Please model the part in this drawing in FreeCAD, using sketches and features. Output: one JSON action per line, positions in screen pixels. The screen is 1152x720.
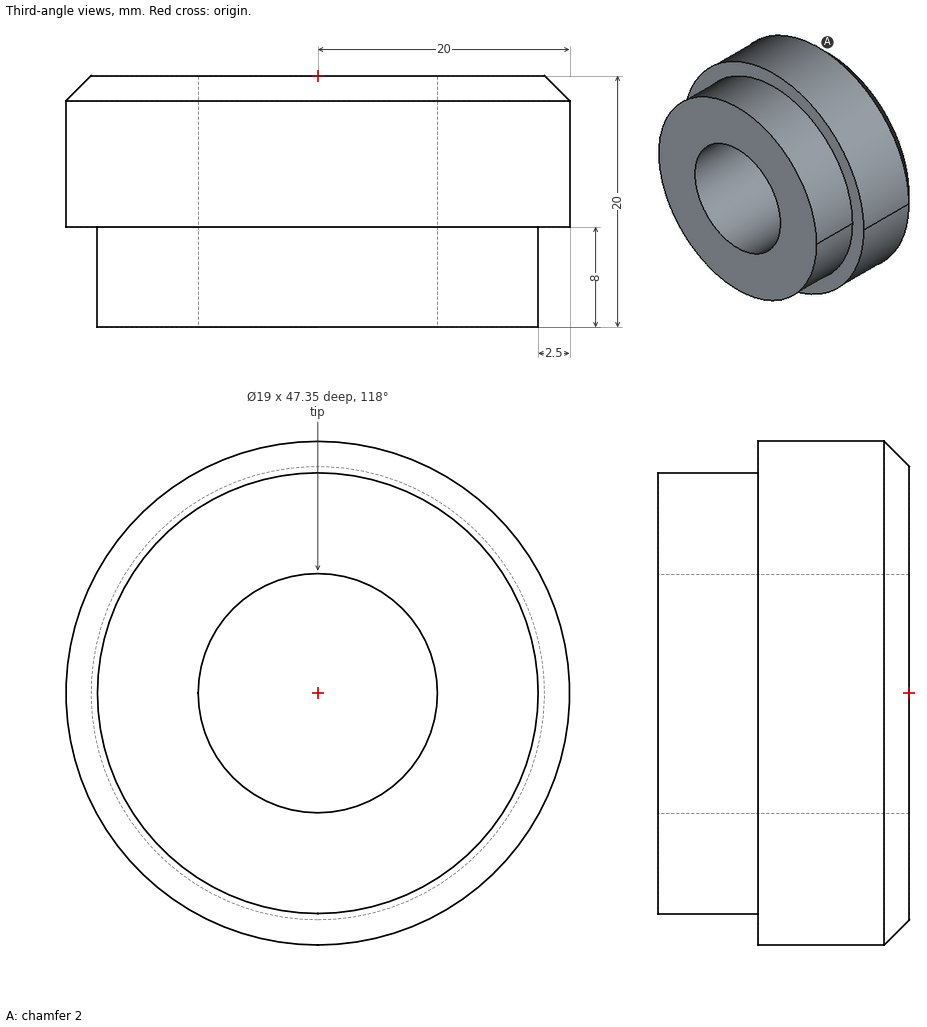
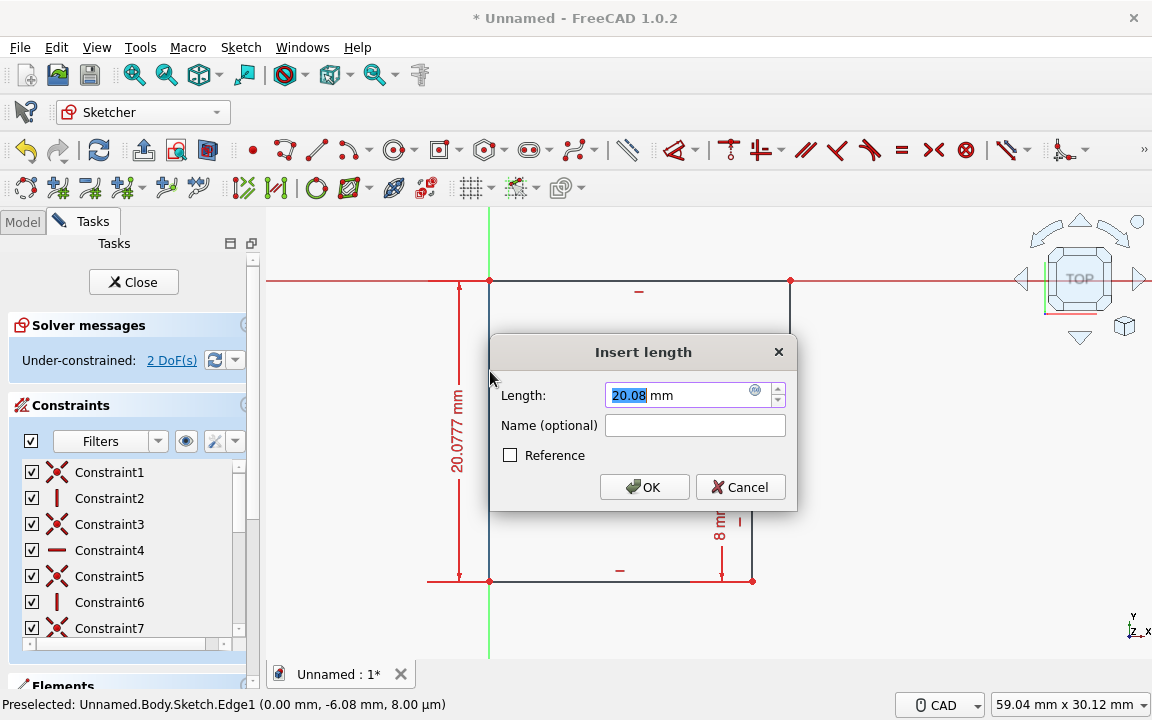
{"action": "type", "text": "20"}
{"action": "key", "text": "Return"}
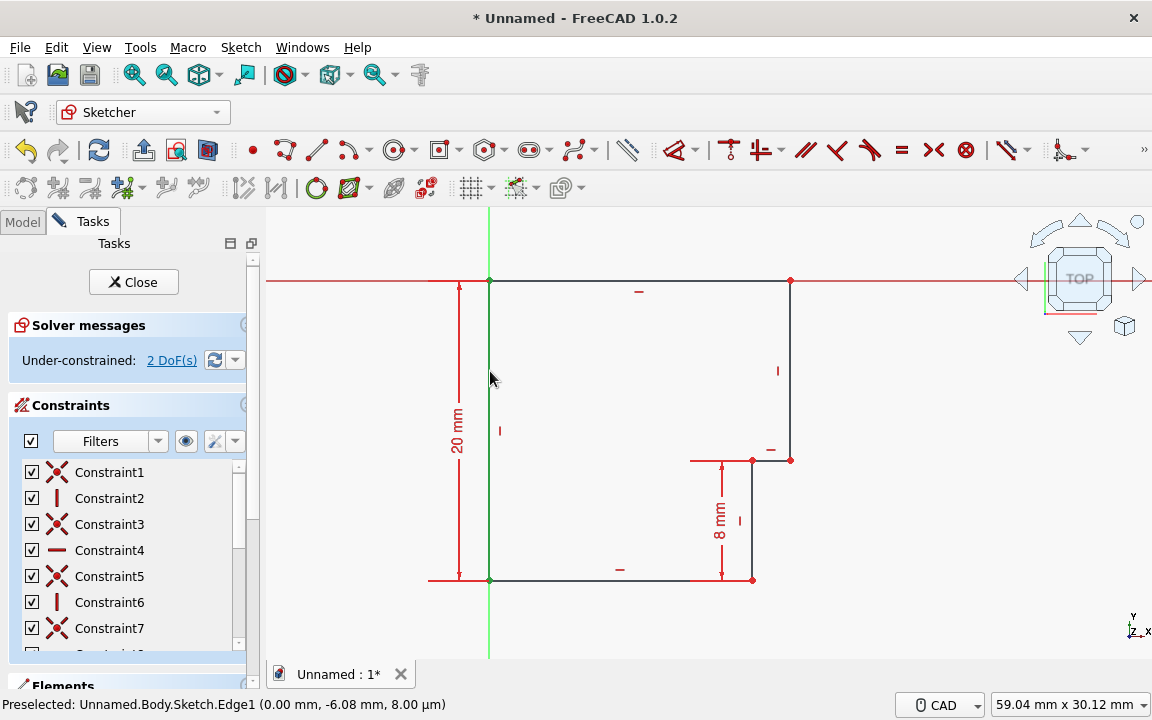
{"action": "left_click", "coordinate": [700, 281]}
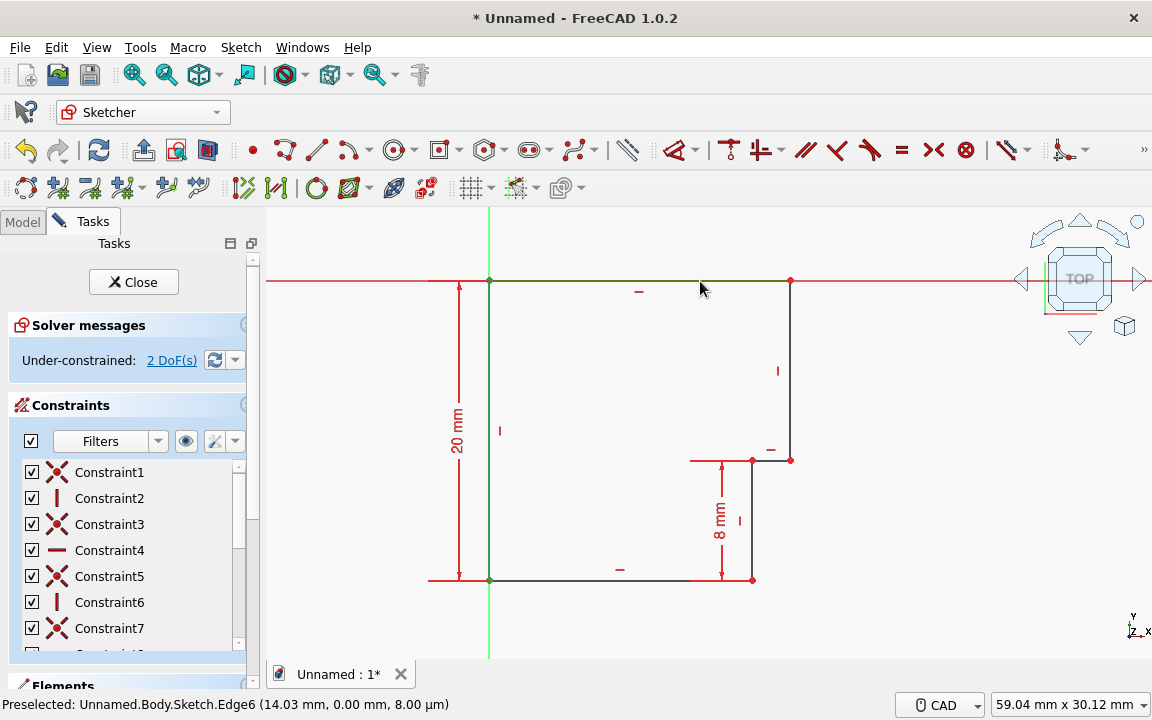
{"action": "key", "text": "l"}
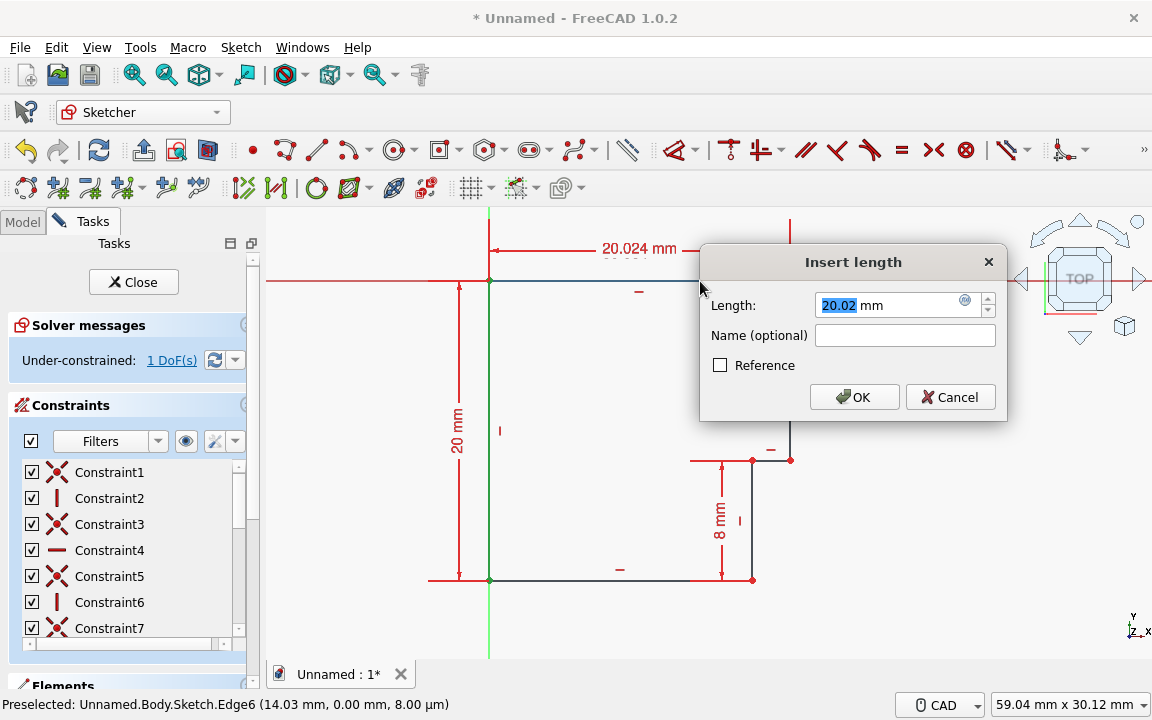
{"action": "type", "text": "20"}
{"action": "key", "text": "Return"}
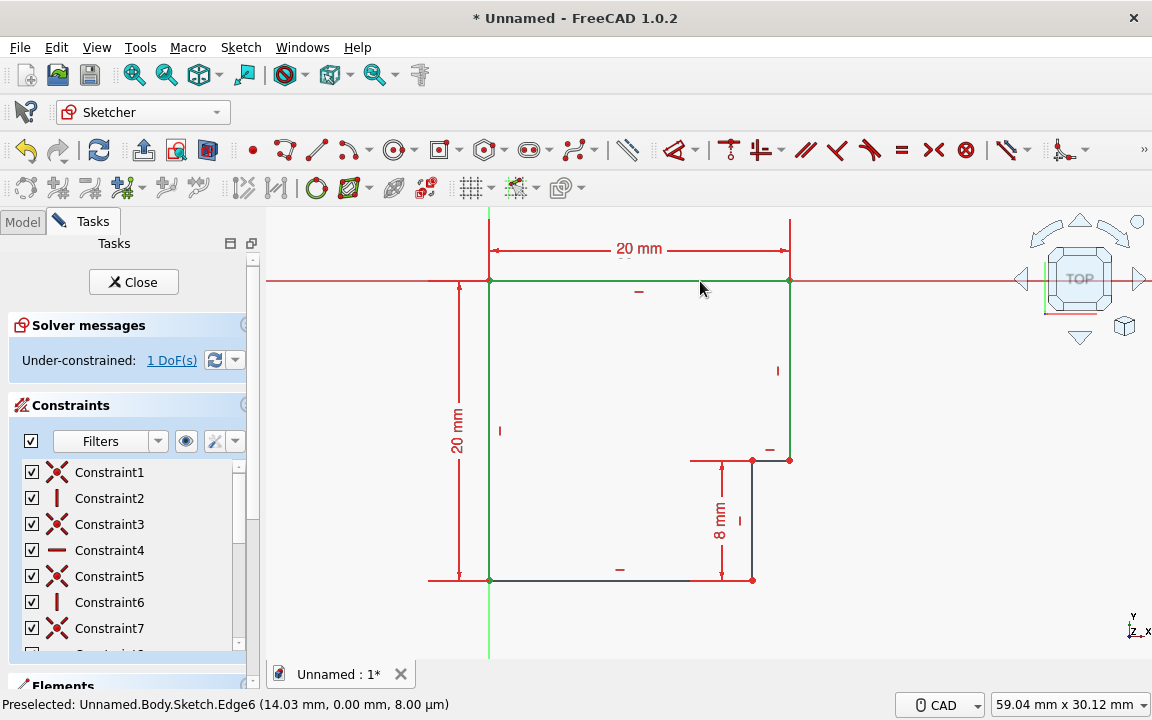
{"action": "scroll", "coordinate": [763, 461], "scroll_direction": "up", "scroll_amount": 2}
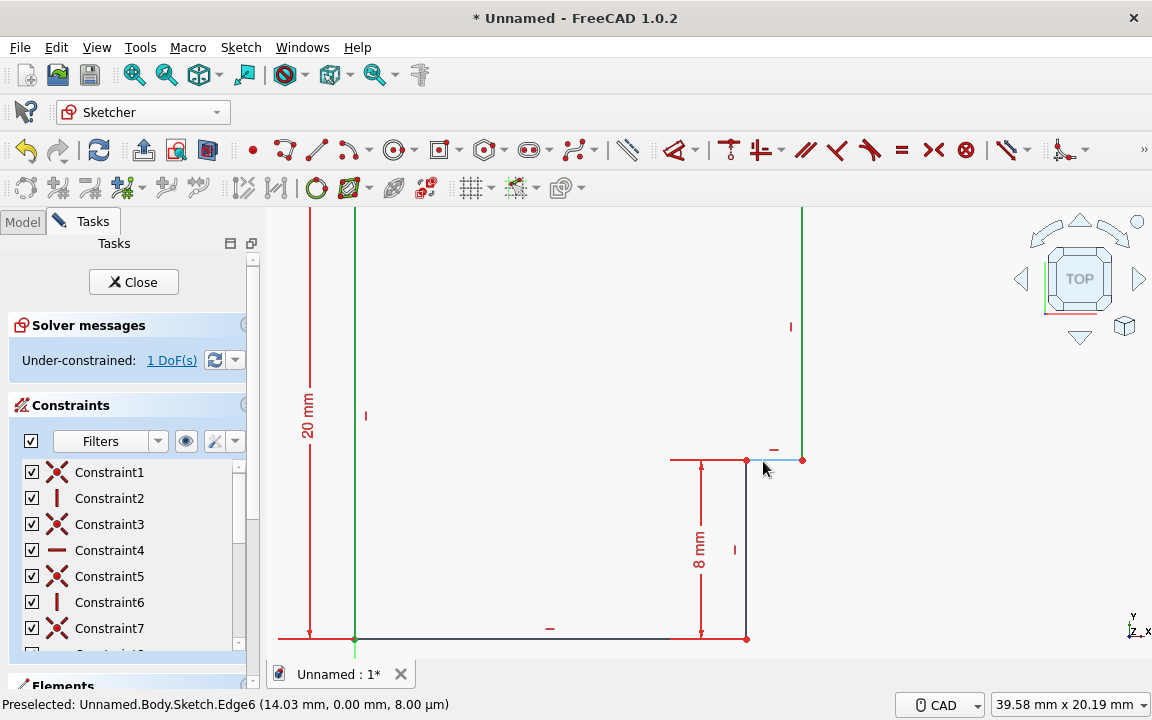
{"action": "left_click", "coordinate": [763, 460]}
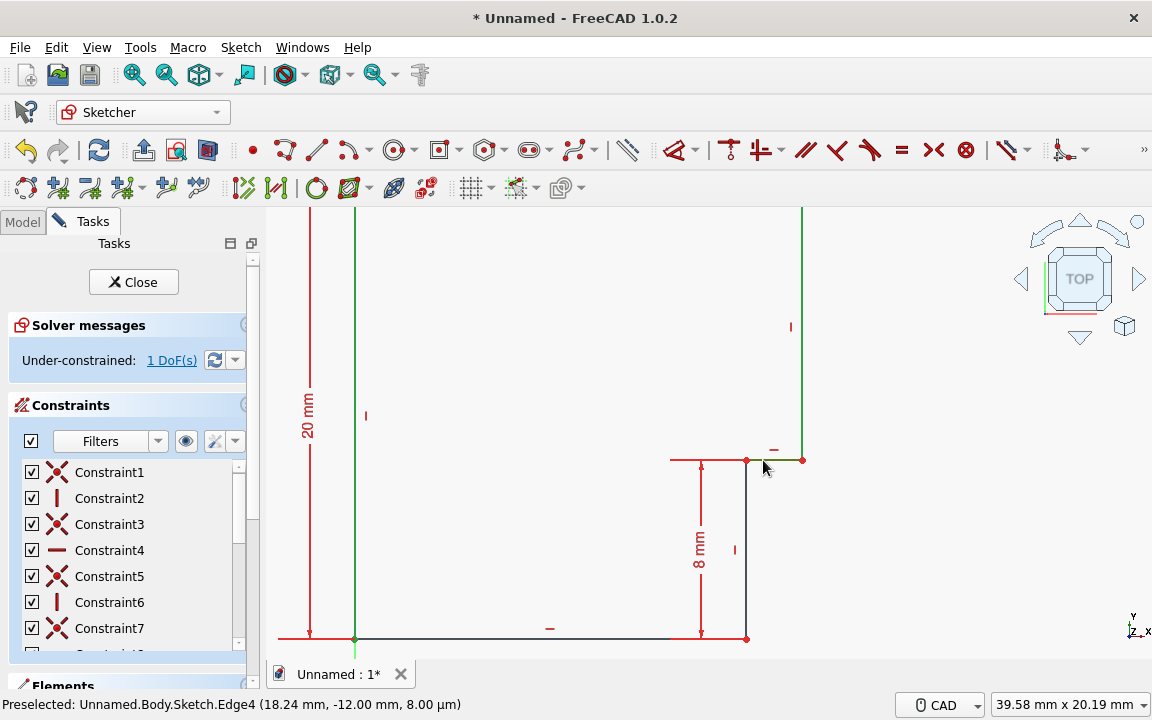
{"action": "left_click", "coordinate": [698, 150]}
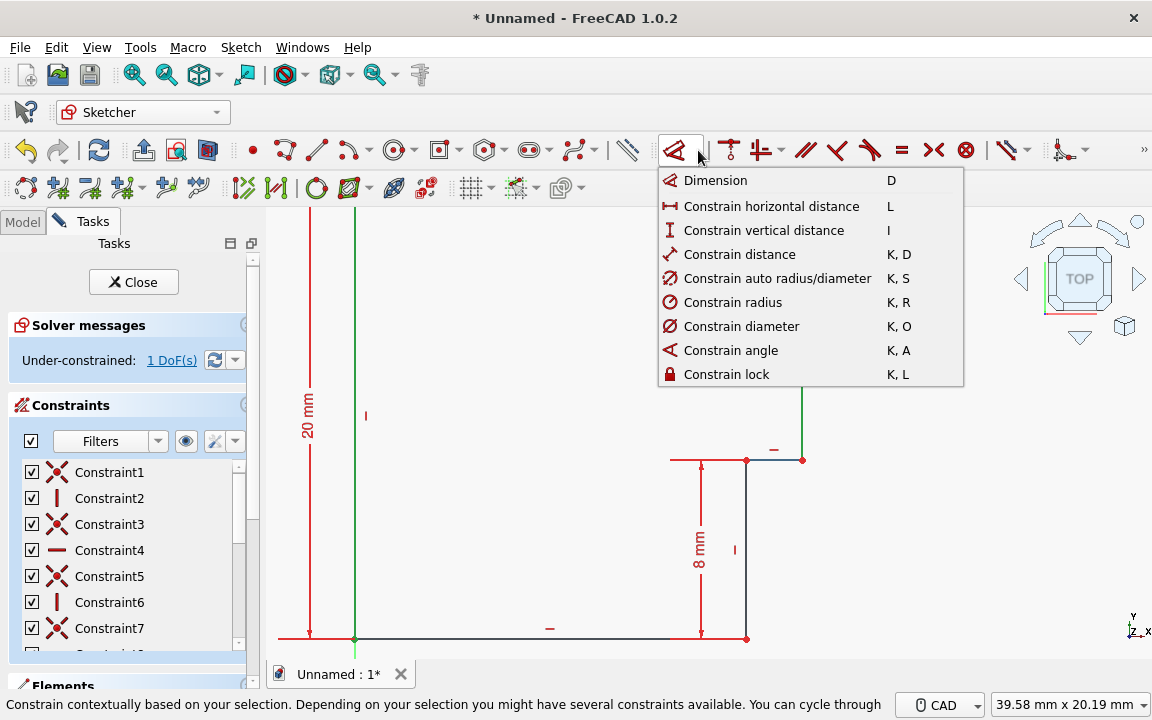
{"action": "left_click", "coordinate": [811, 206]}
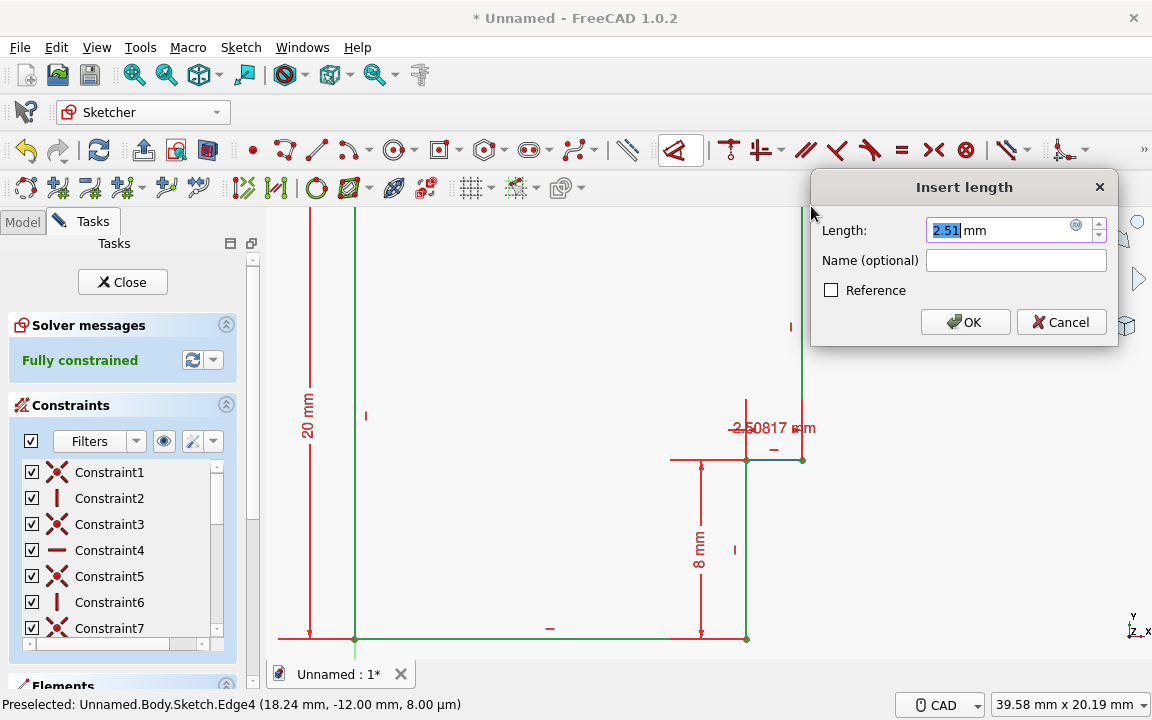
{"action": "type", "text": "2.5"}
{"action": "key", "text": "Return"}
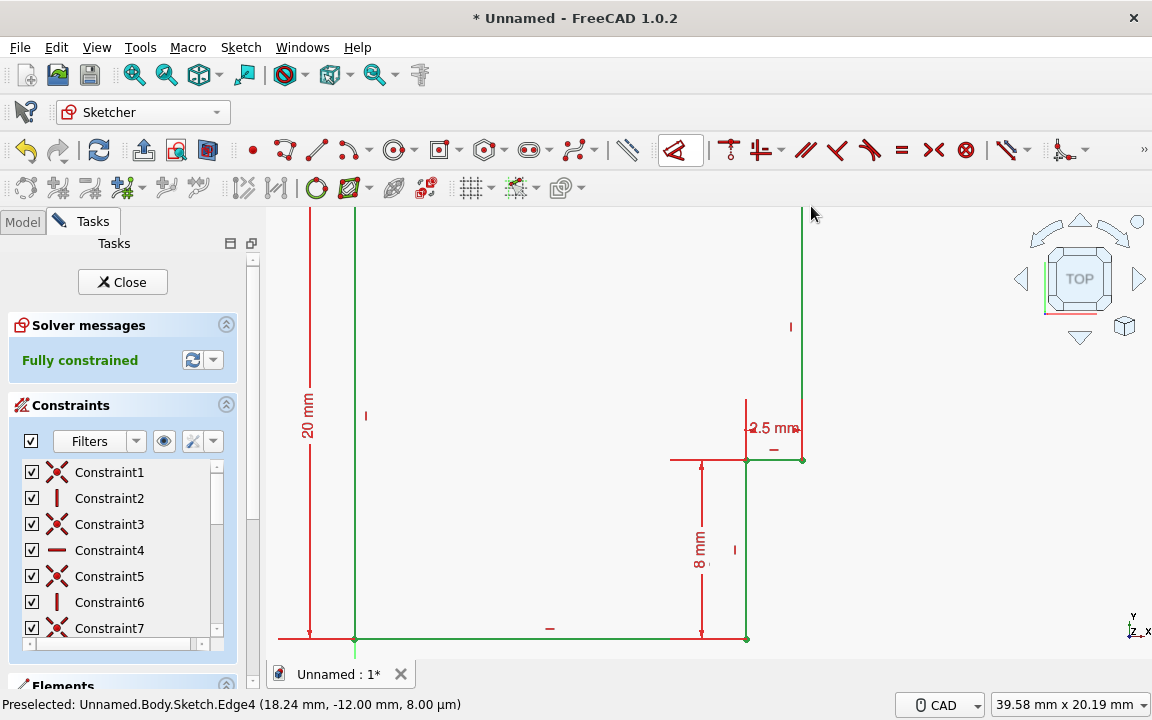
{"action": "left_click", "coordinate": [123, 282]}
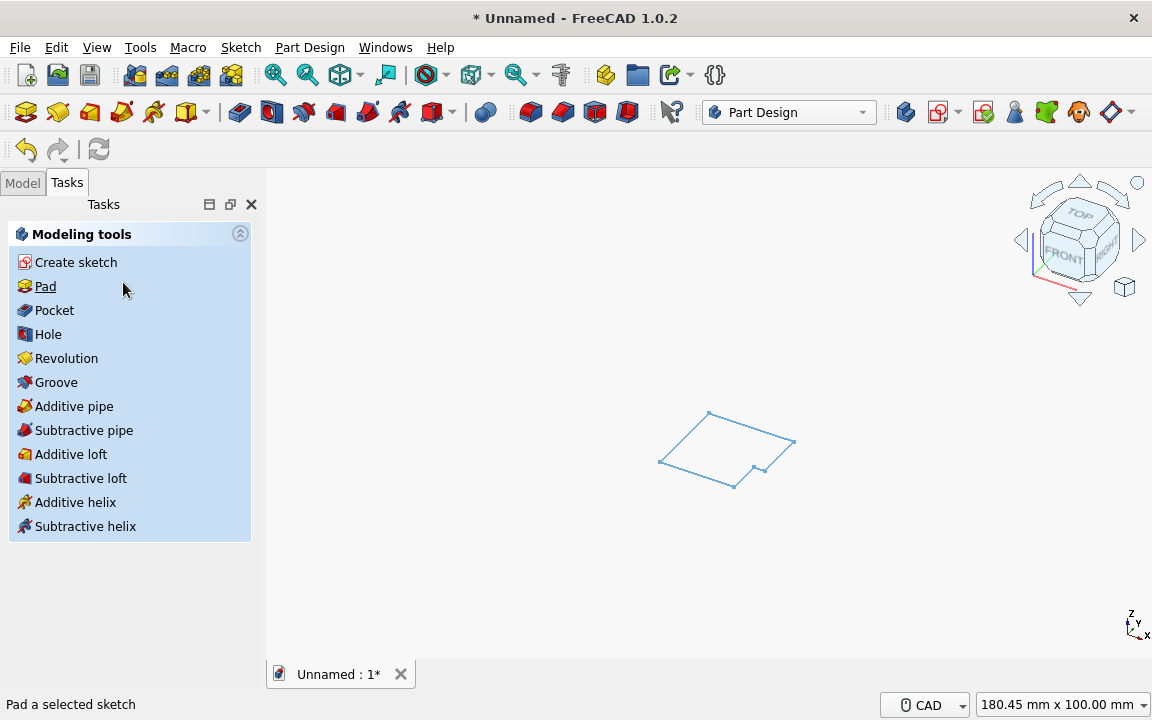
{"action": "left_click", "coordinate": [58, 112]}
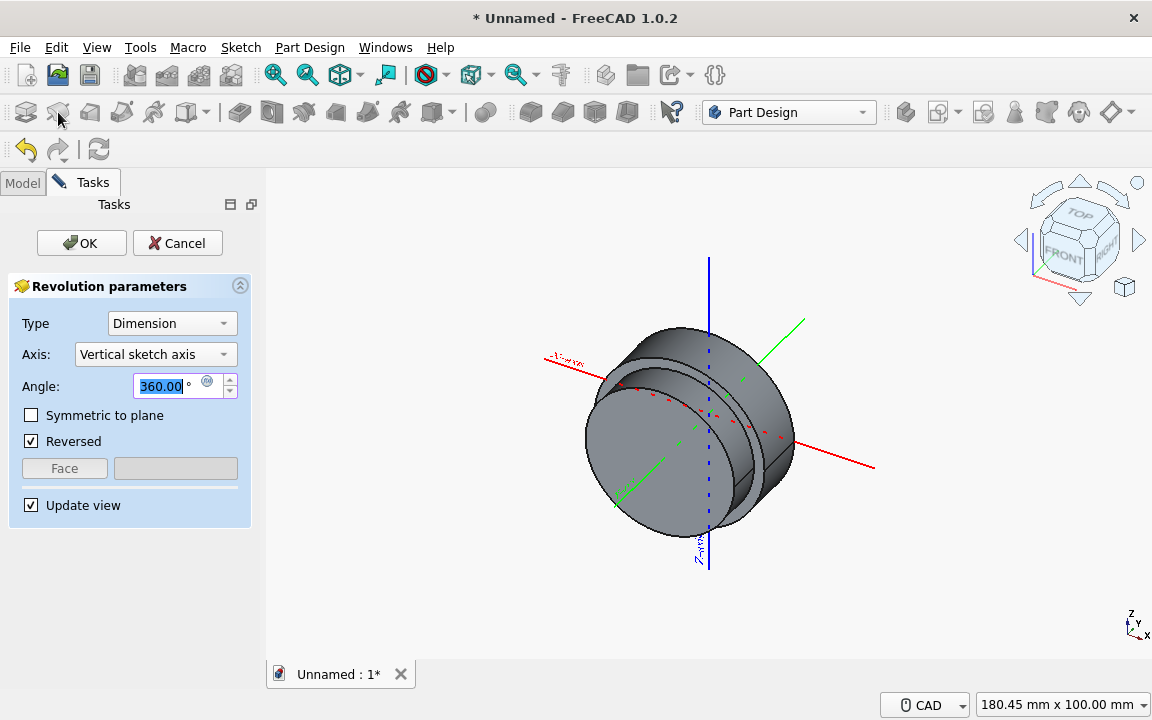
{"action": "left_click", "coordinate": [82, 243]}